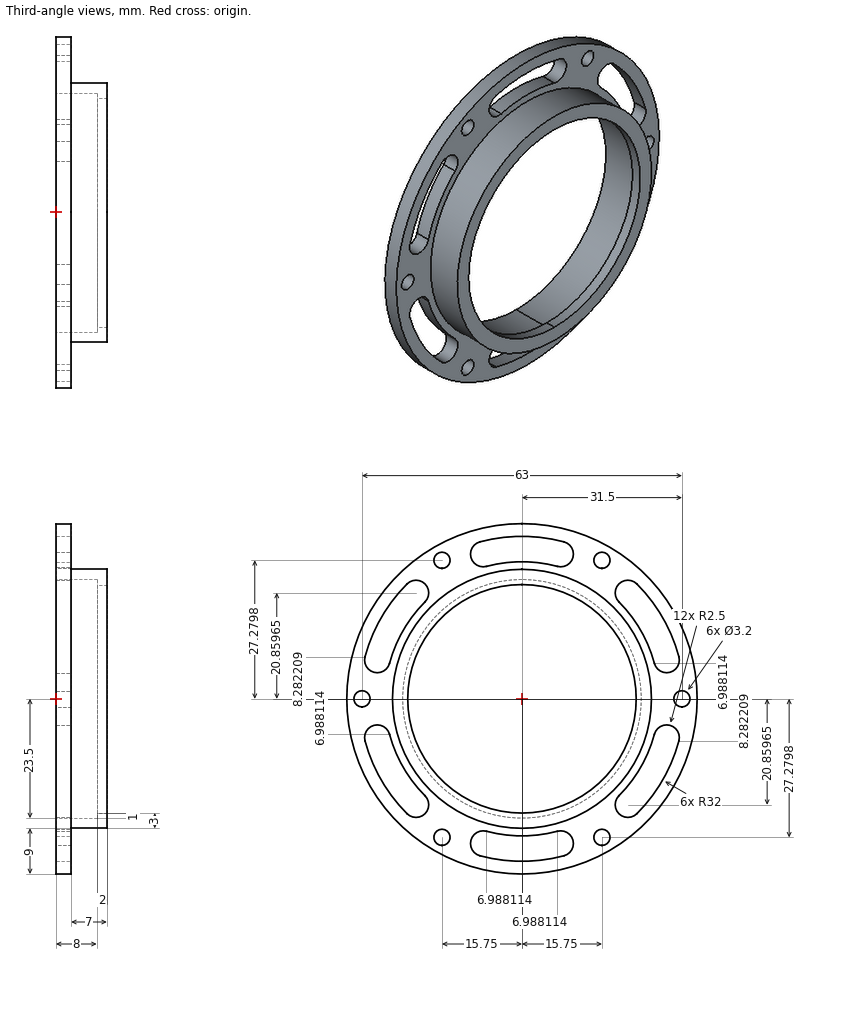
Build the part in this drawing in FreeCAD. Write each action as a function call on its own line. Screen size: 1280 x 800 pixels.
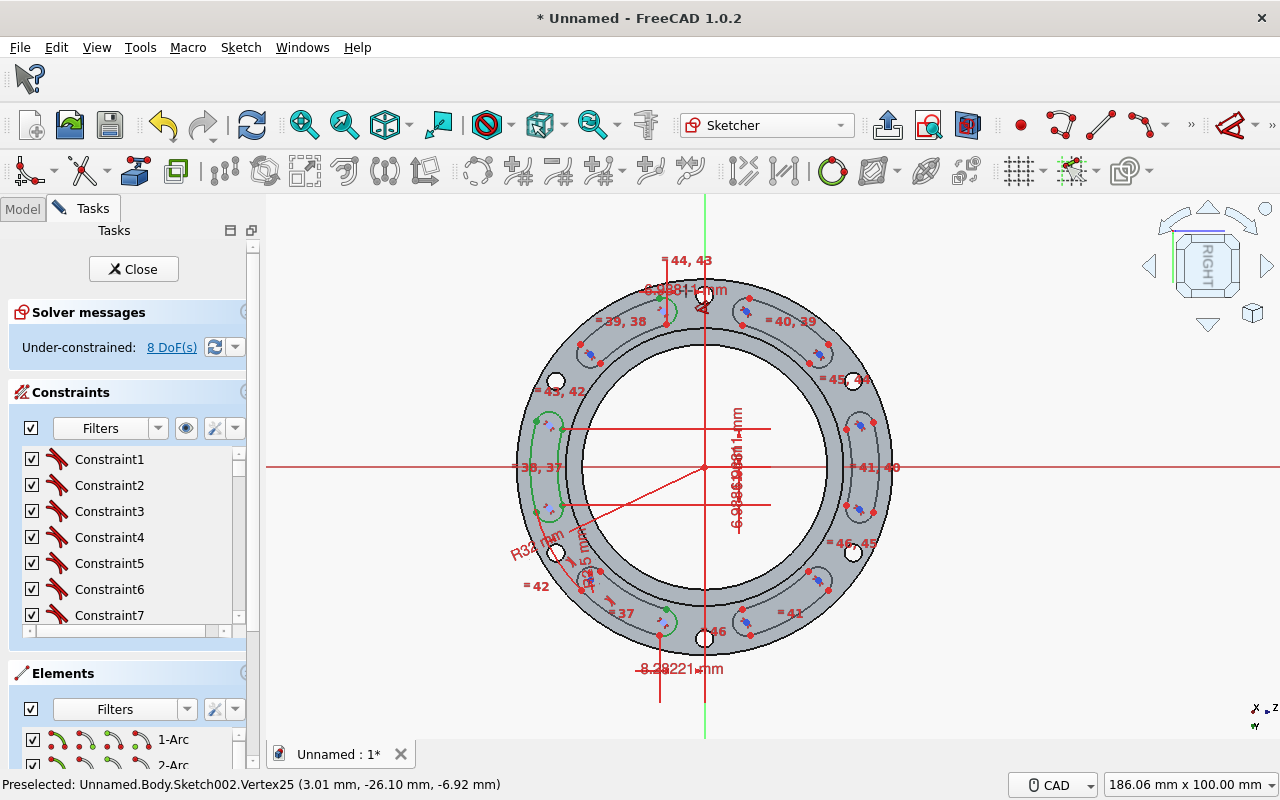
click(750, 299)
click(727, 265)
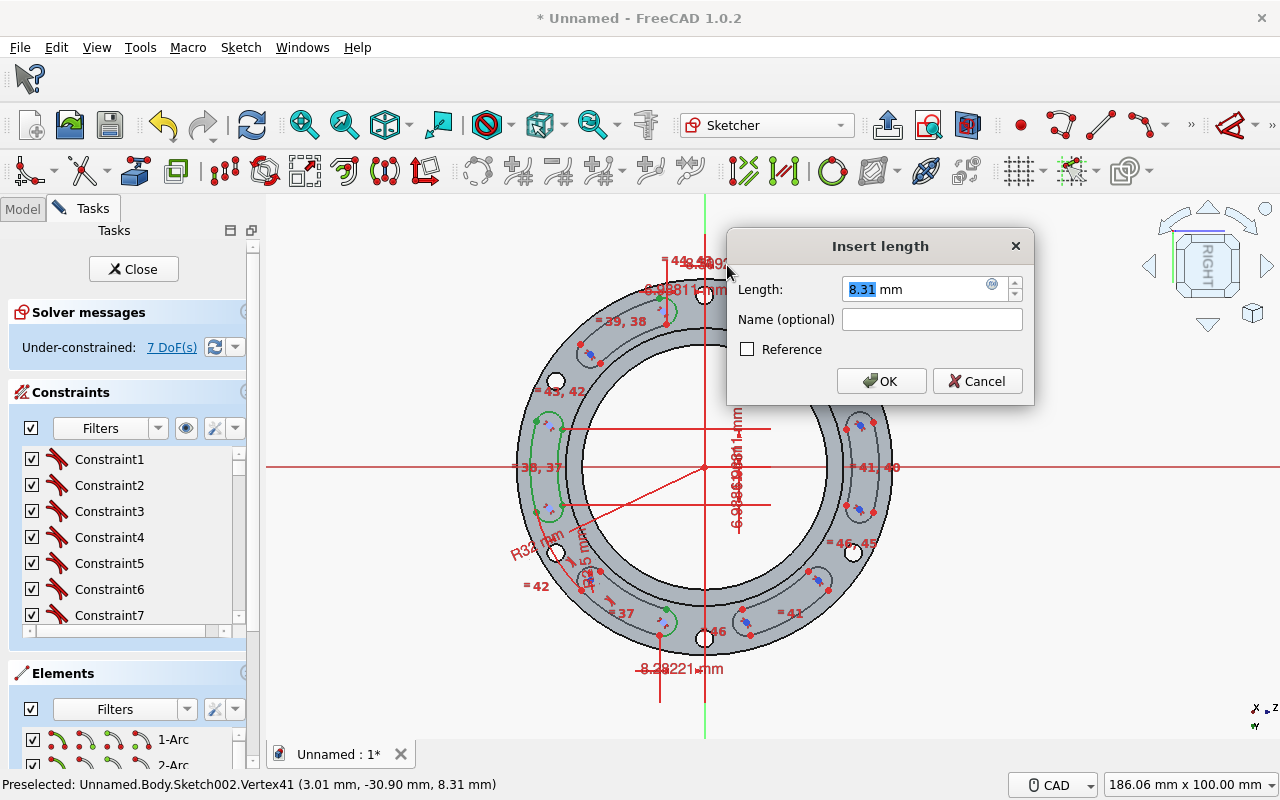
text(8.282209)
key(Return)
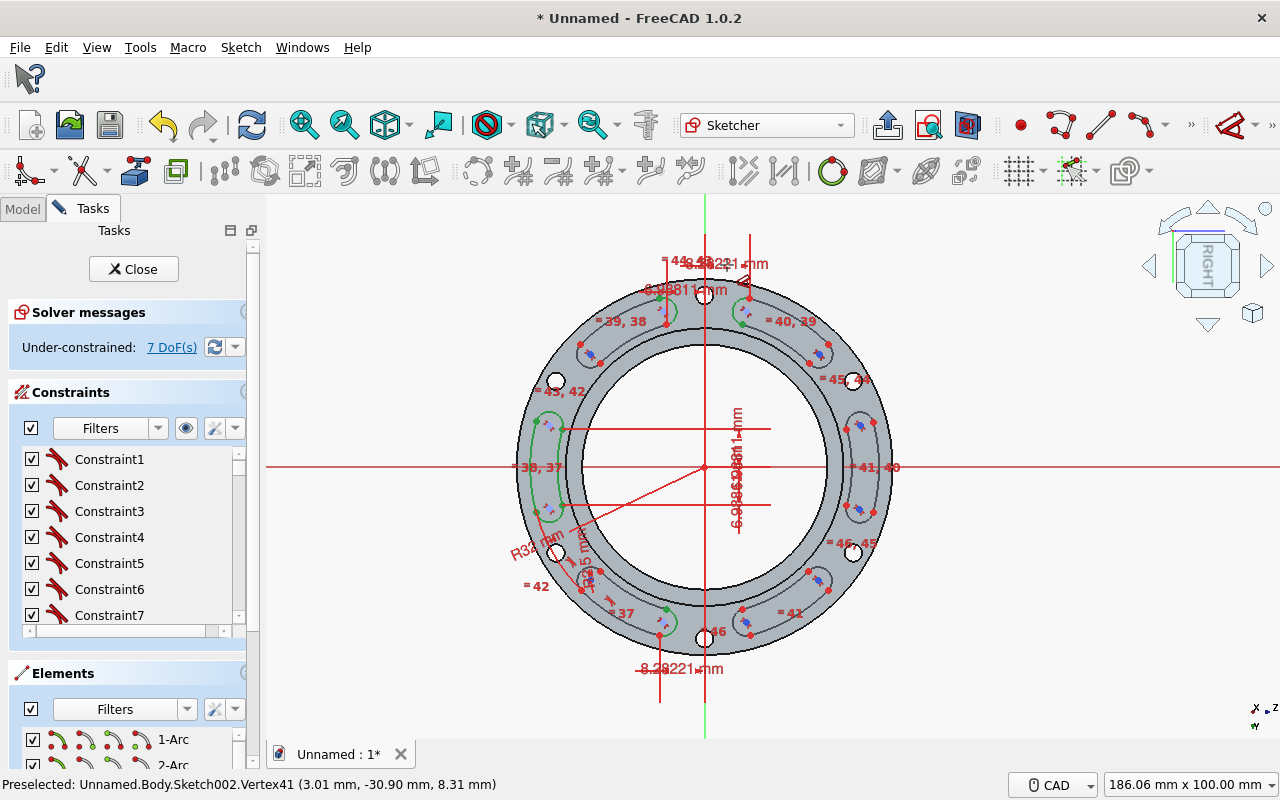
click(847, 506)
click(905, 486)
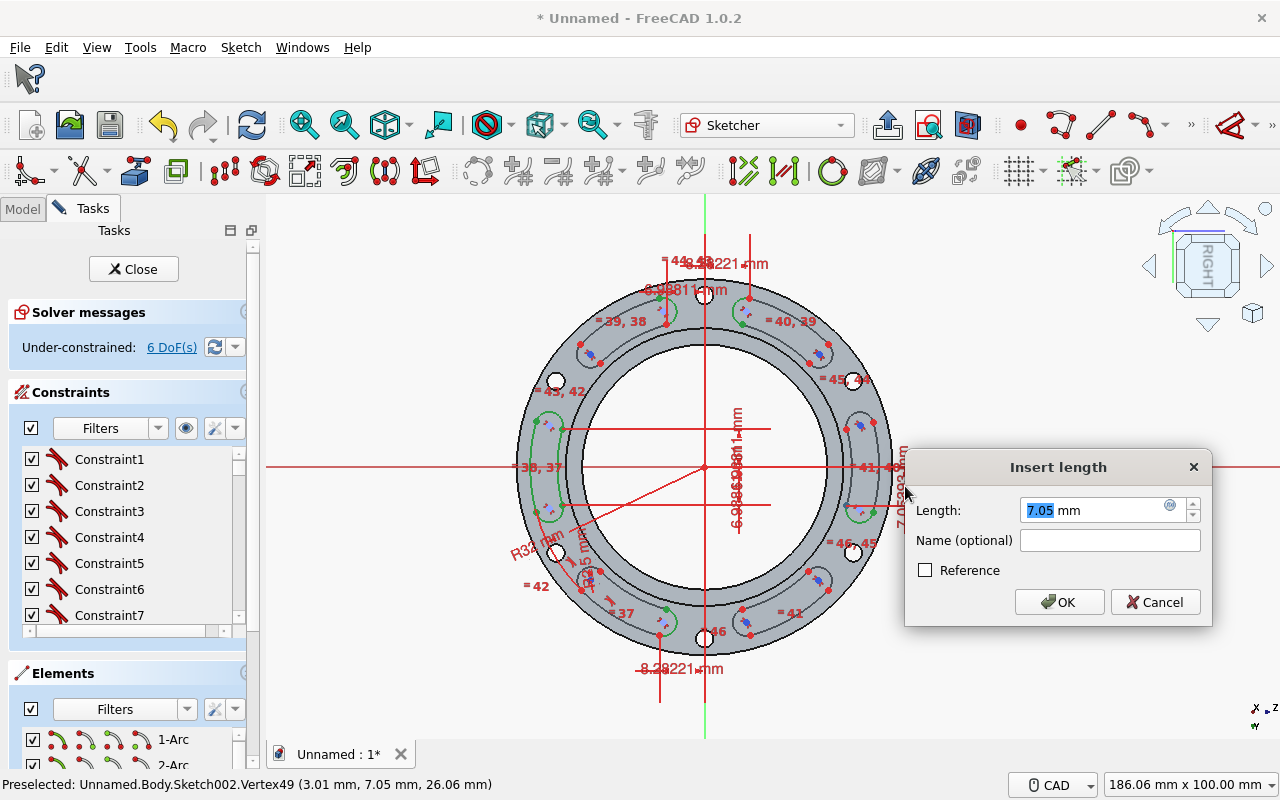
text(6.988114)
key(Return)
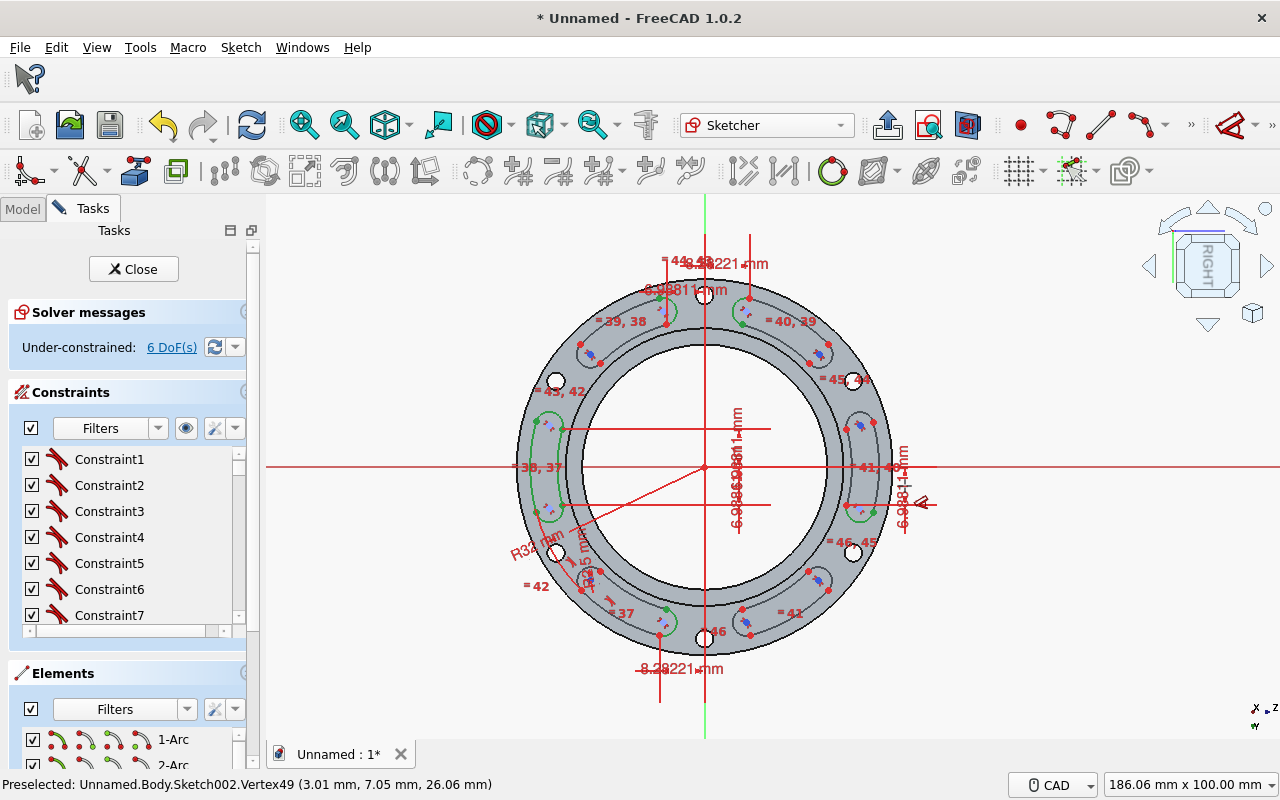
click(847, 429)
click(905, 448)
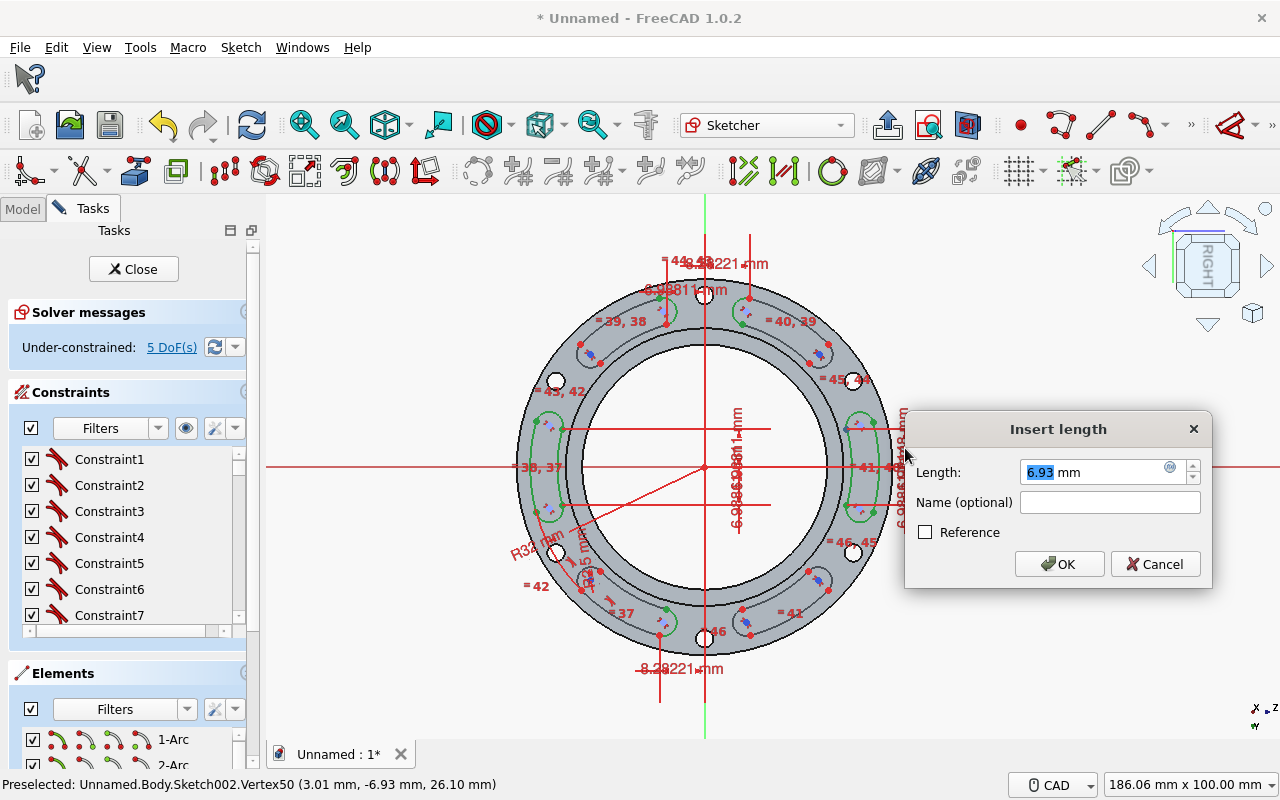
text(6.988114)
key(Return)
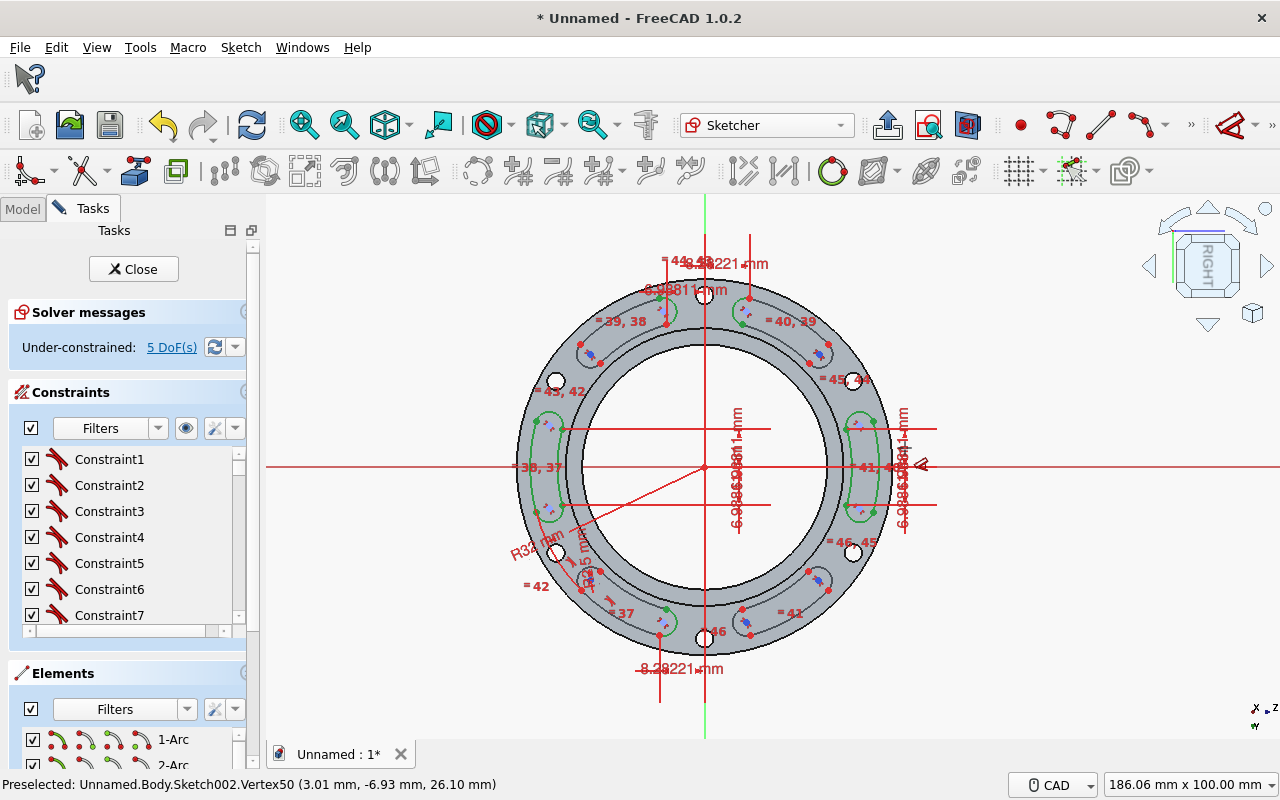
click(743, 609)
click(724, 643)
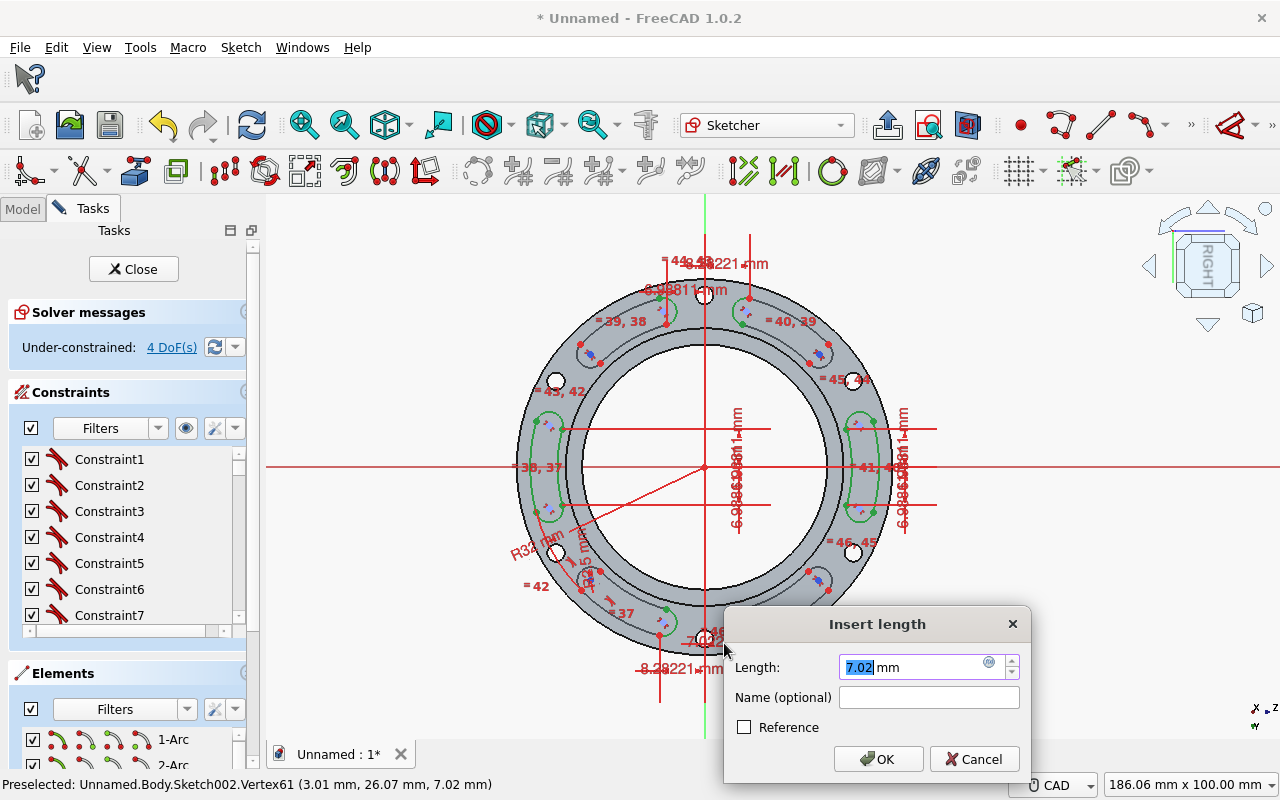
text(6.988114)
key(Return)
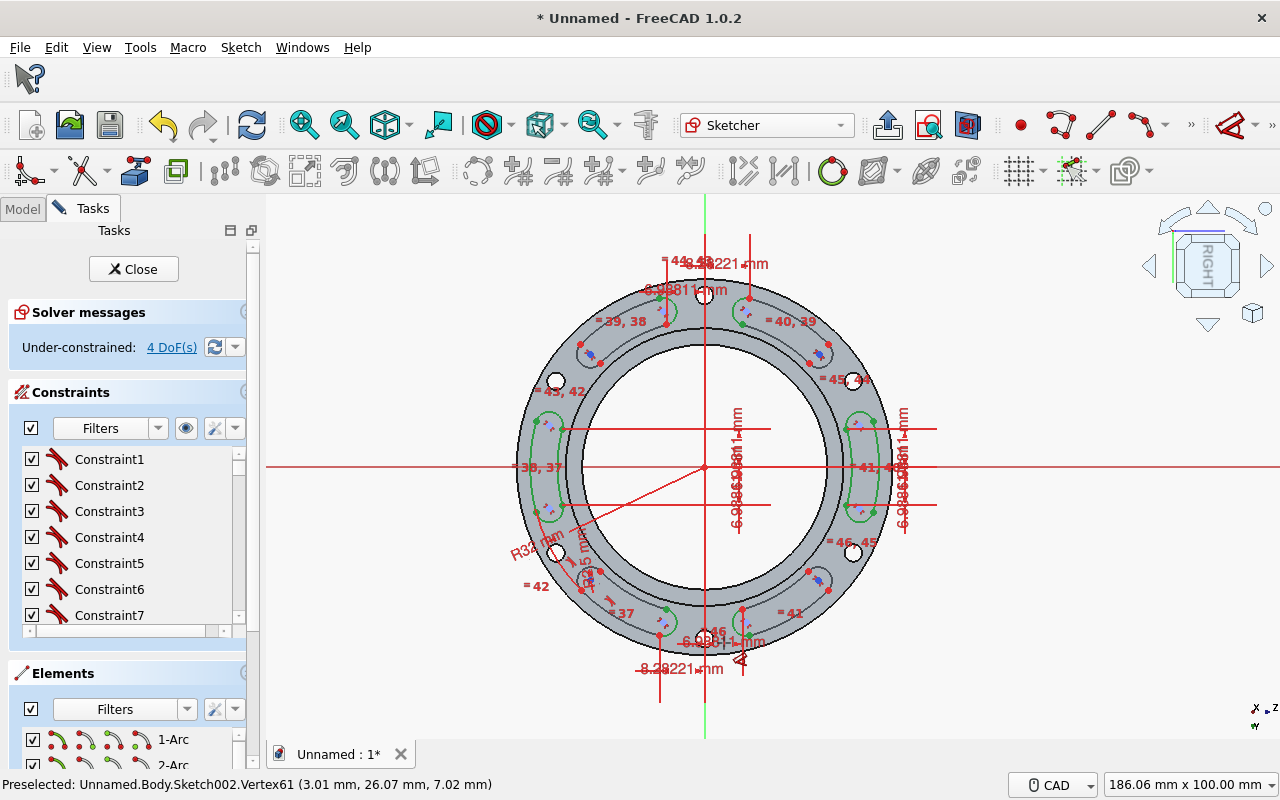
click(591, 581)
click(648, 433)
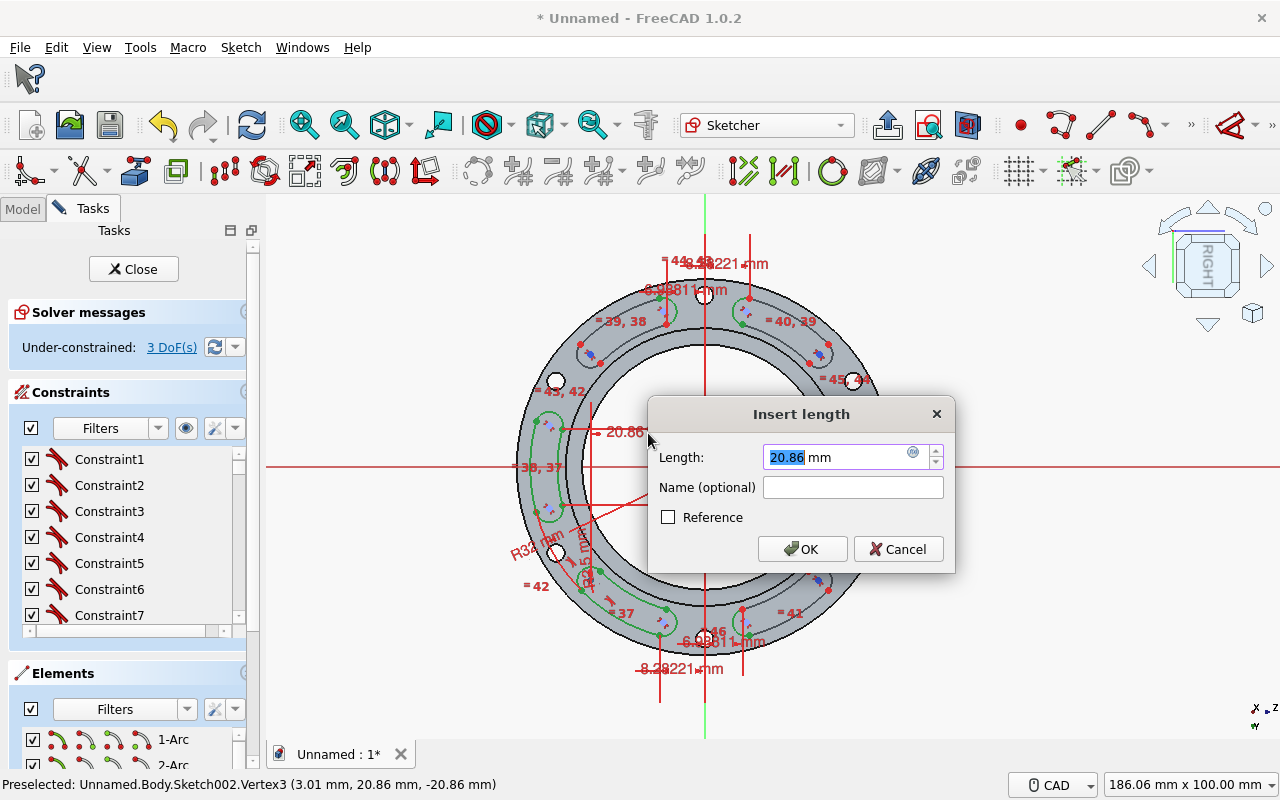
text(20.85965)
key(Return)